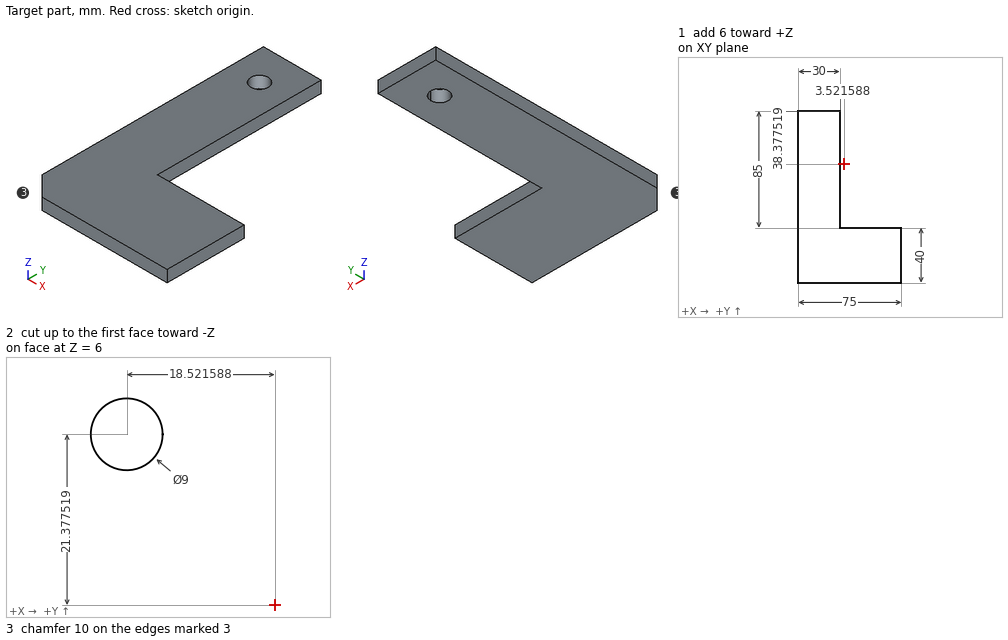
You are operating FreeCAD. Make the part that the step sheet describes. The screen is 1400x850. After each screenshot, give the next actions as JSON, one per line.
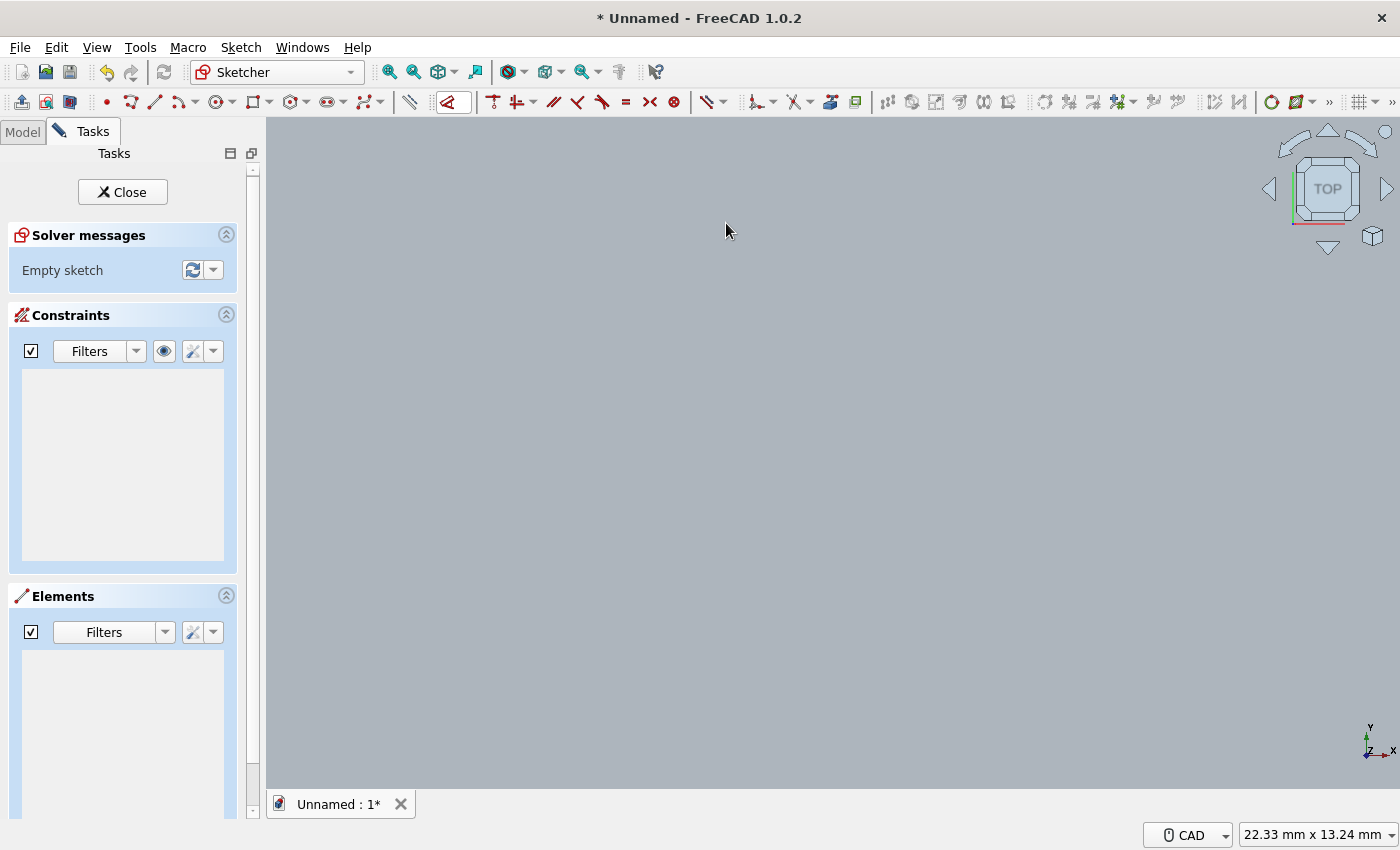
{"action": "left_click", "coordinate": [216, 102]}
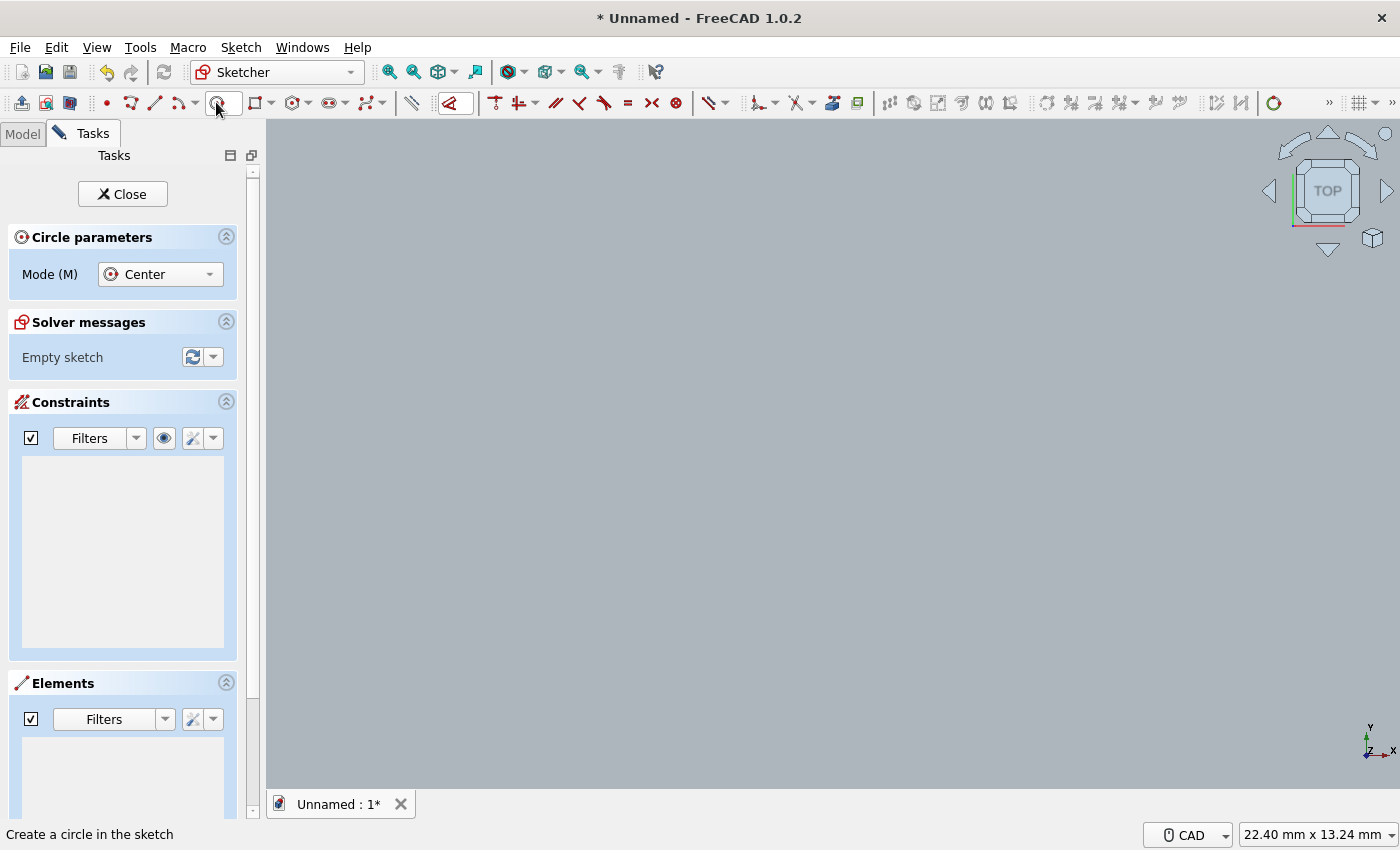
{"action": "left_click", "coordinate": [759, 448]}
{"action": "left_click", "coordinate": [920, 287]}
{"action": "key", "text": "Escape"}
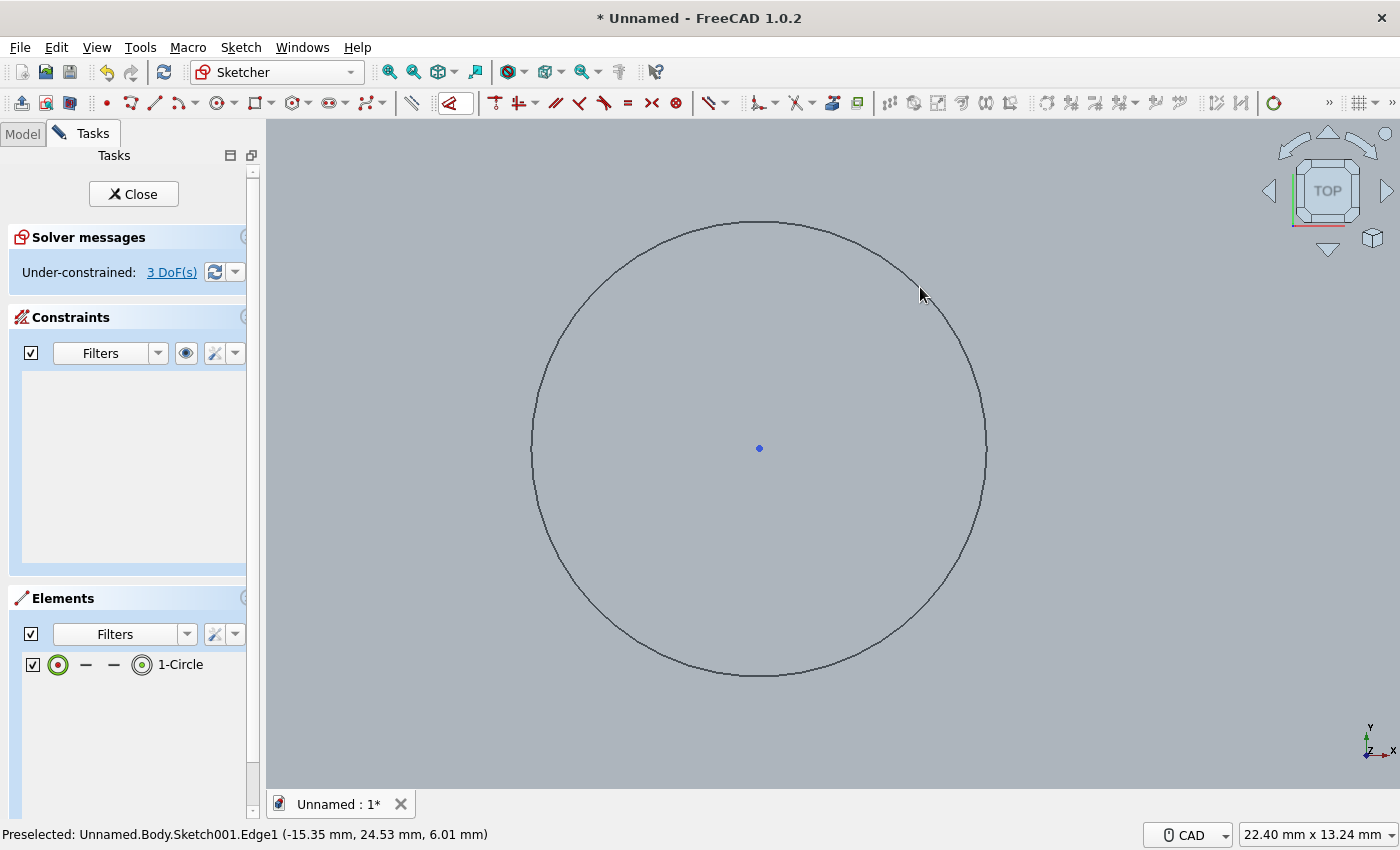
{"action": "left_click", "coordinate": [920, 288]}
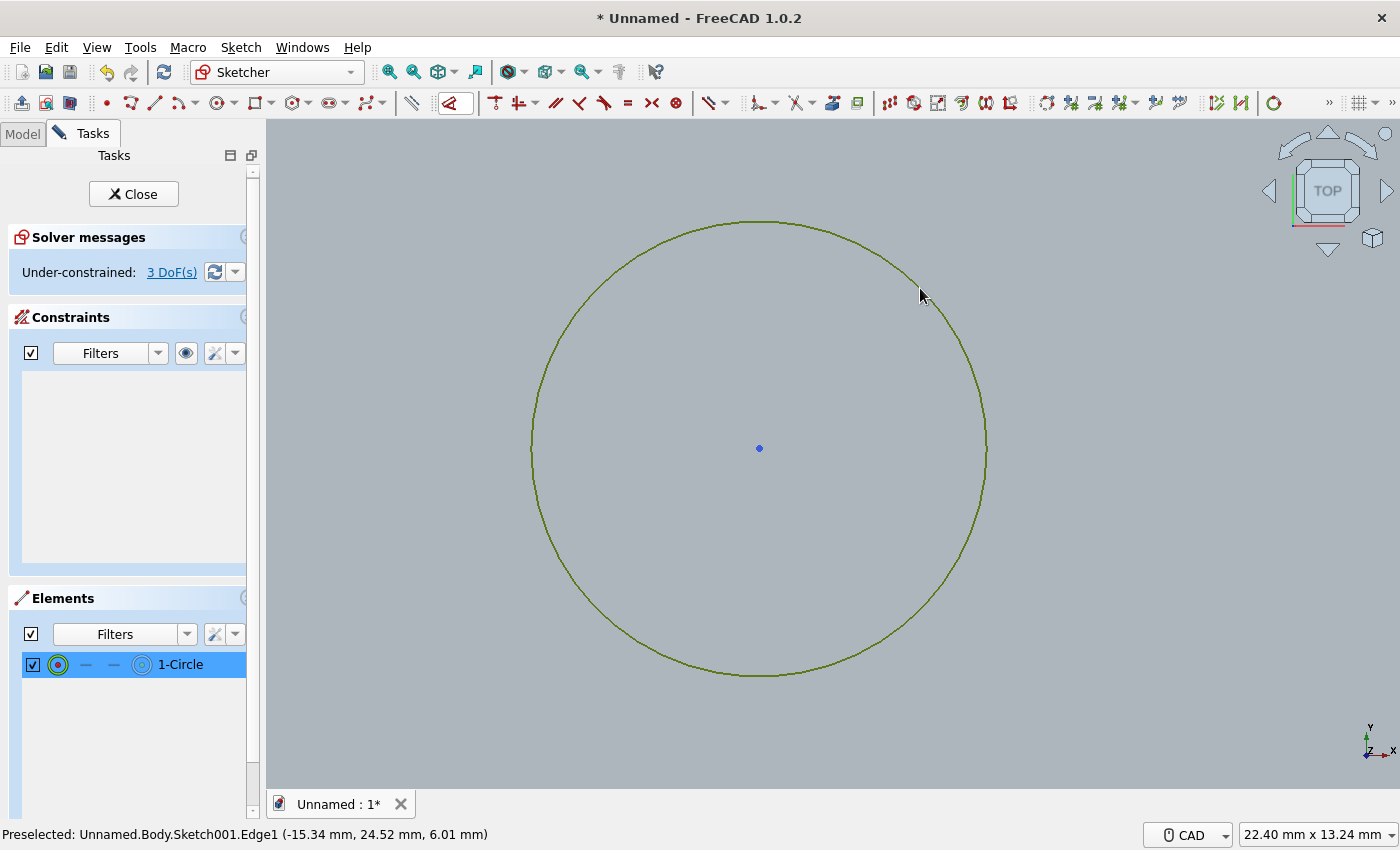
{"action": "key", "text": "k o"}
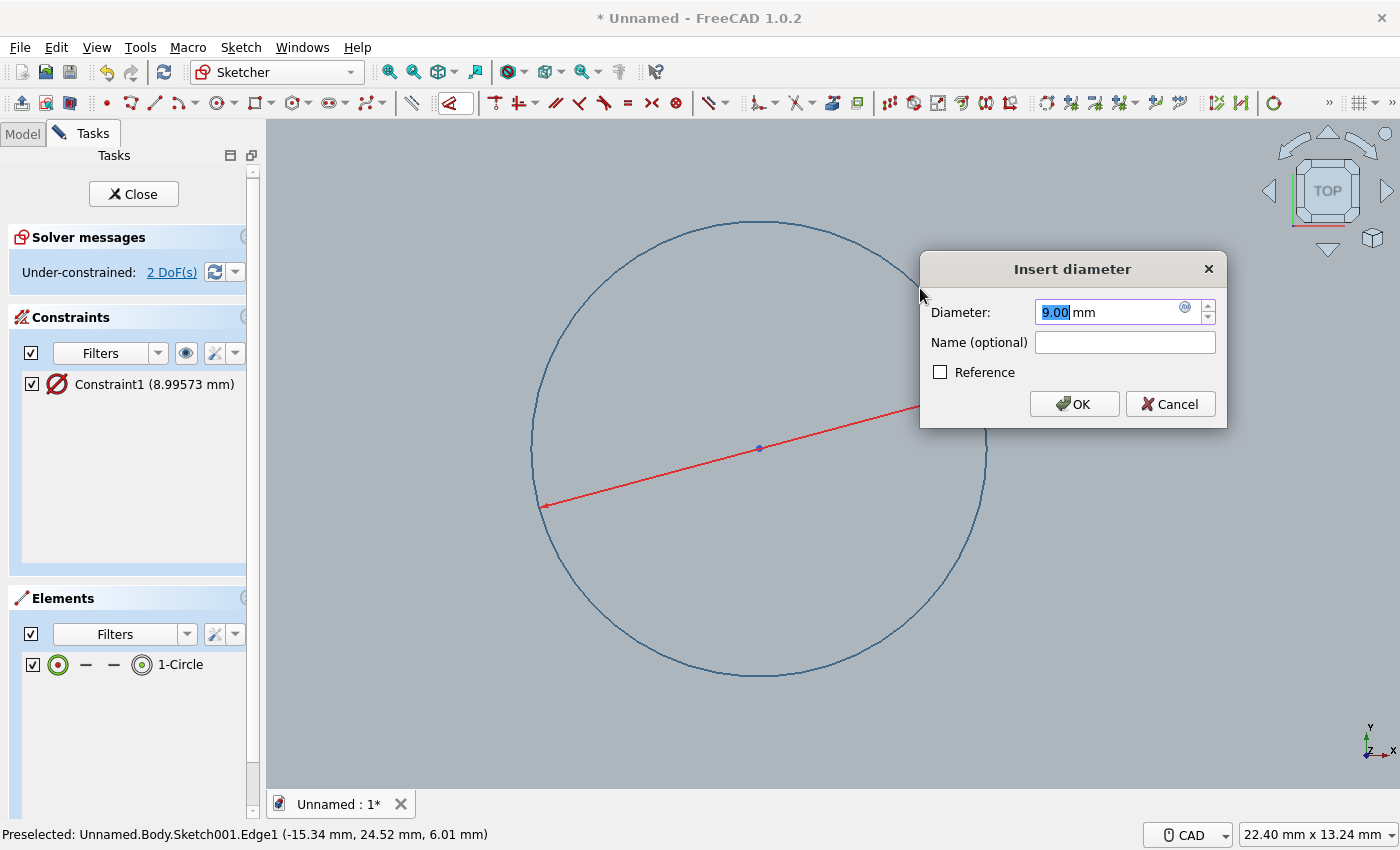
{"action": "type", "text": "9"}
{"action": "key", "text": "Return"}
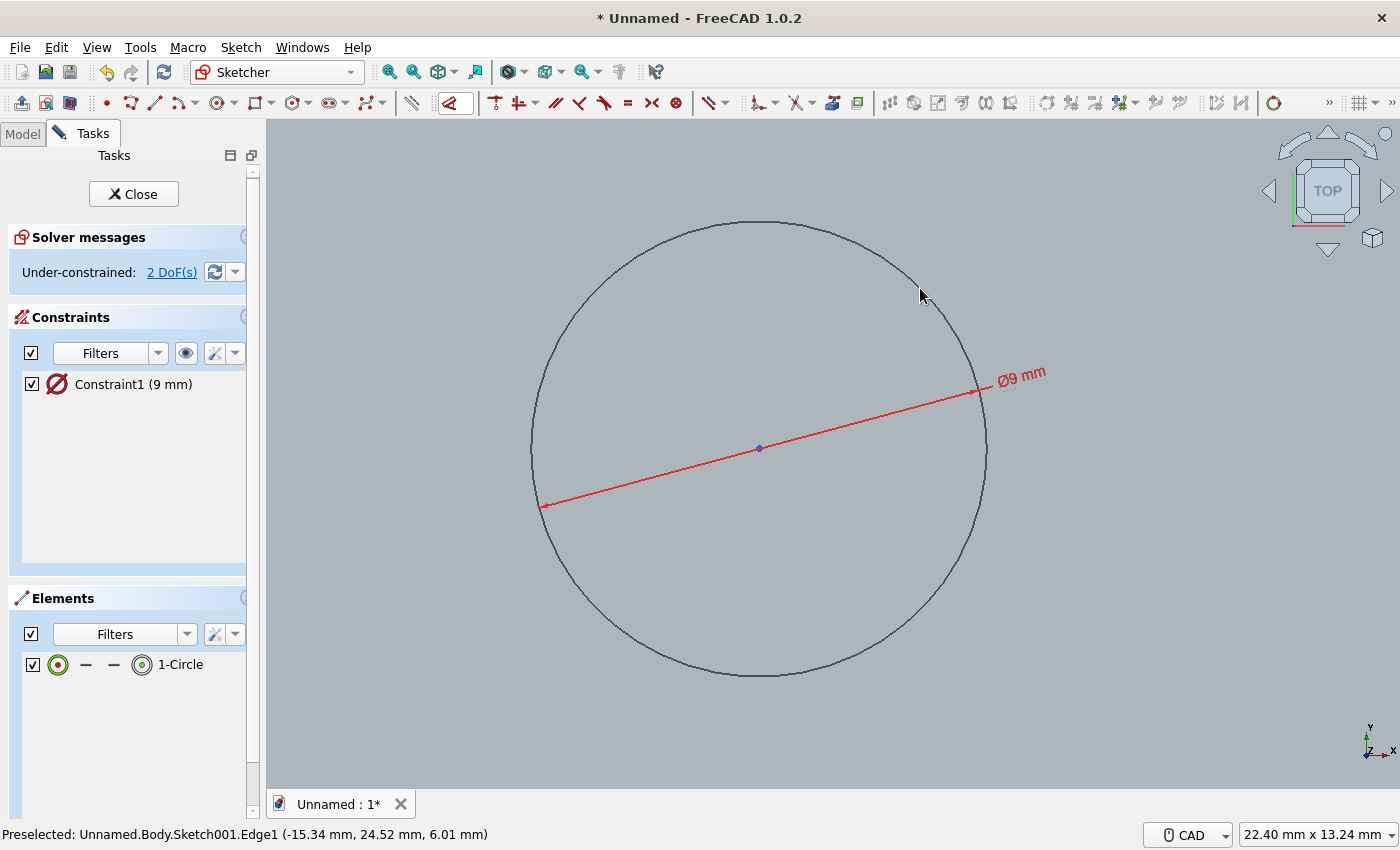
{"action": "left_click", "coordinate": [759, 449]}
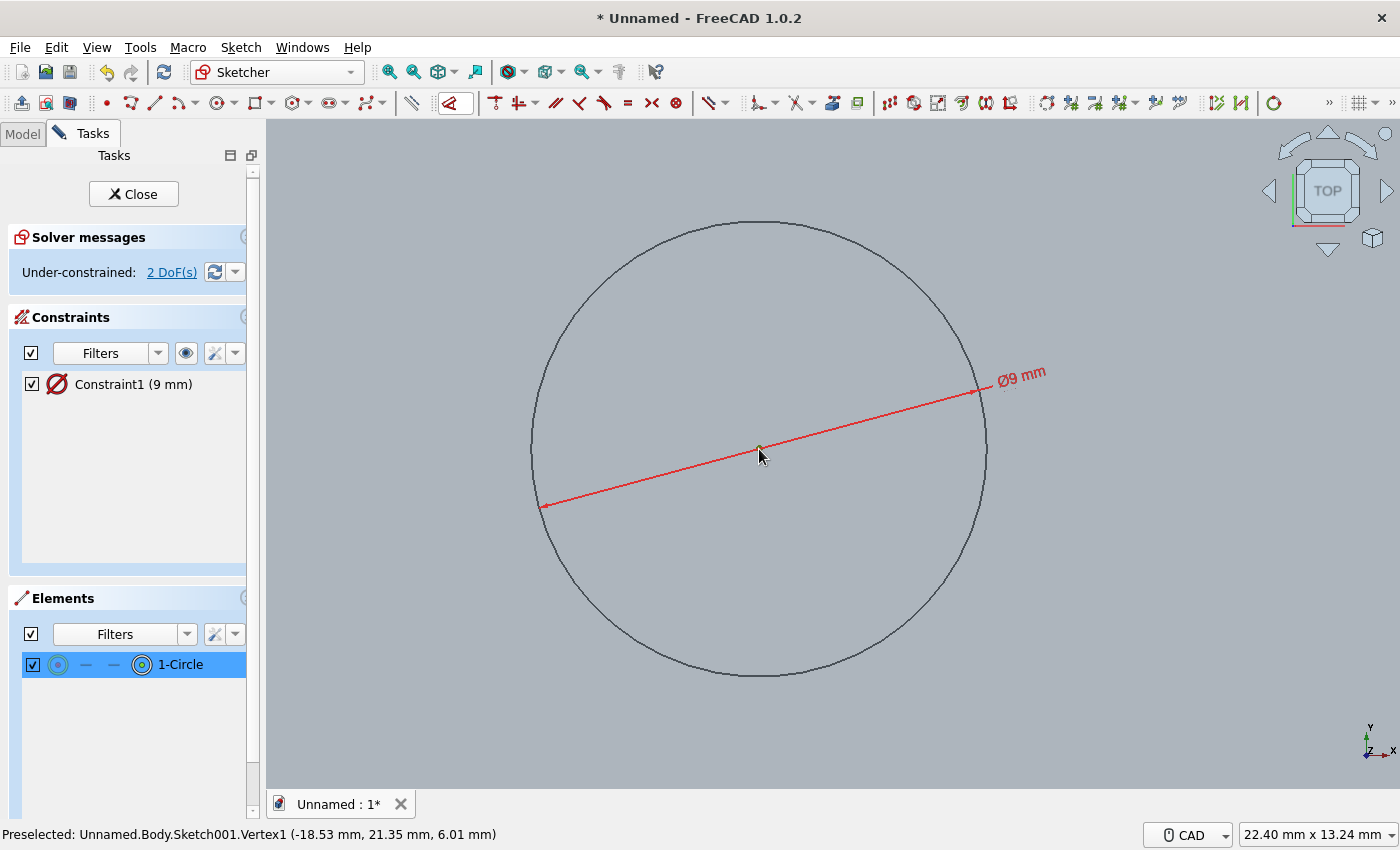
{"action": "left_click", "coordinate": [468, 104]}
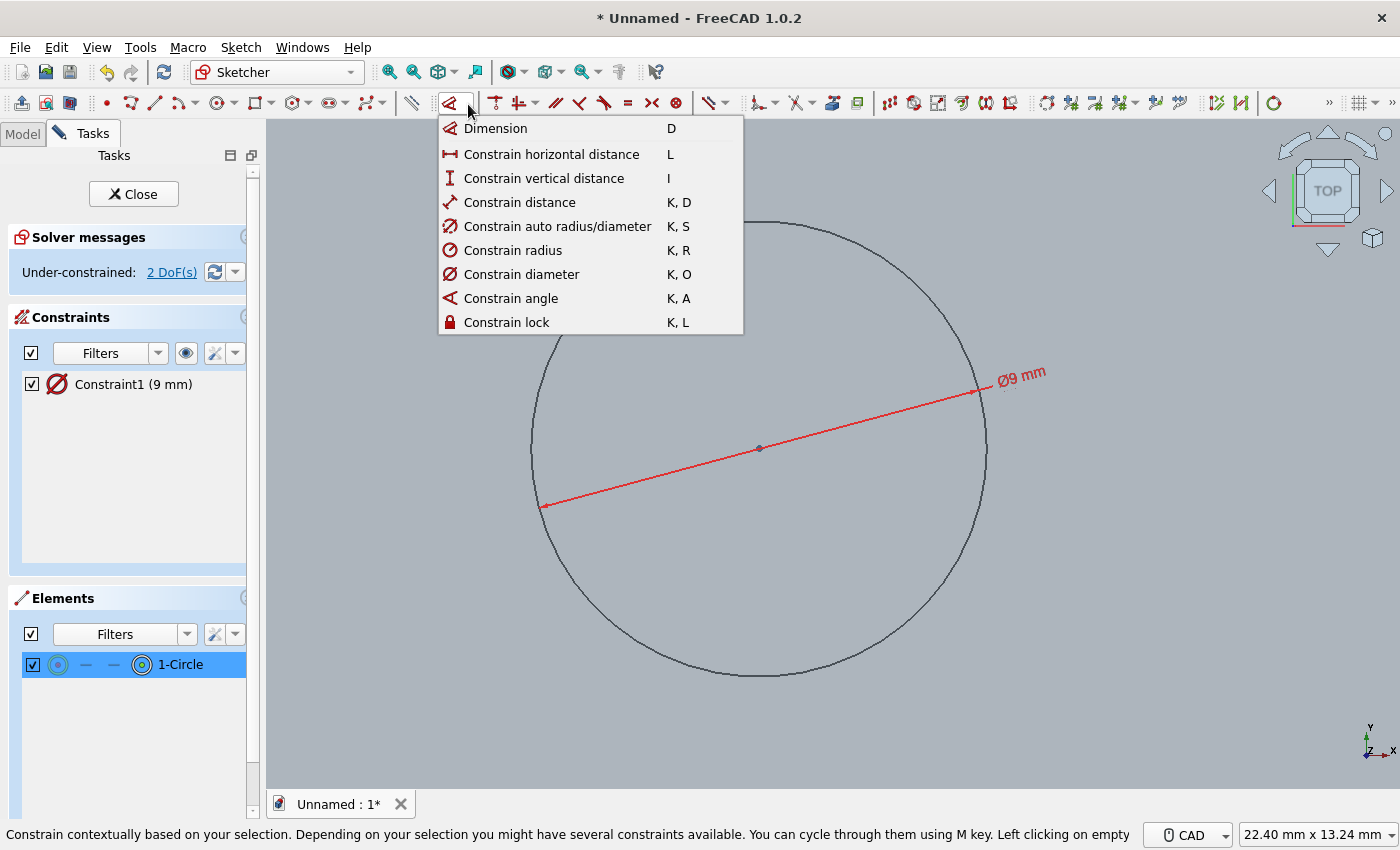
{"action": "left_click", "coordinate": [591, 154]}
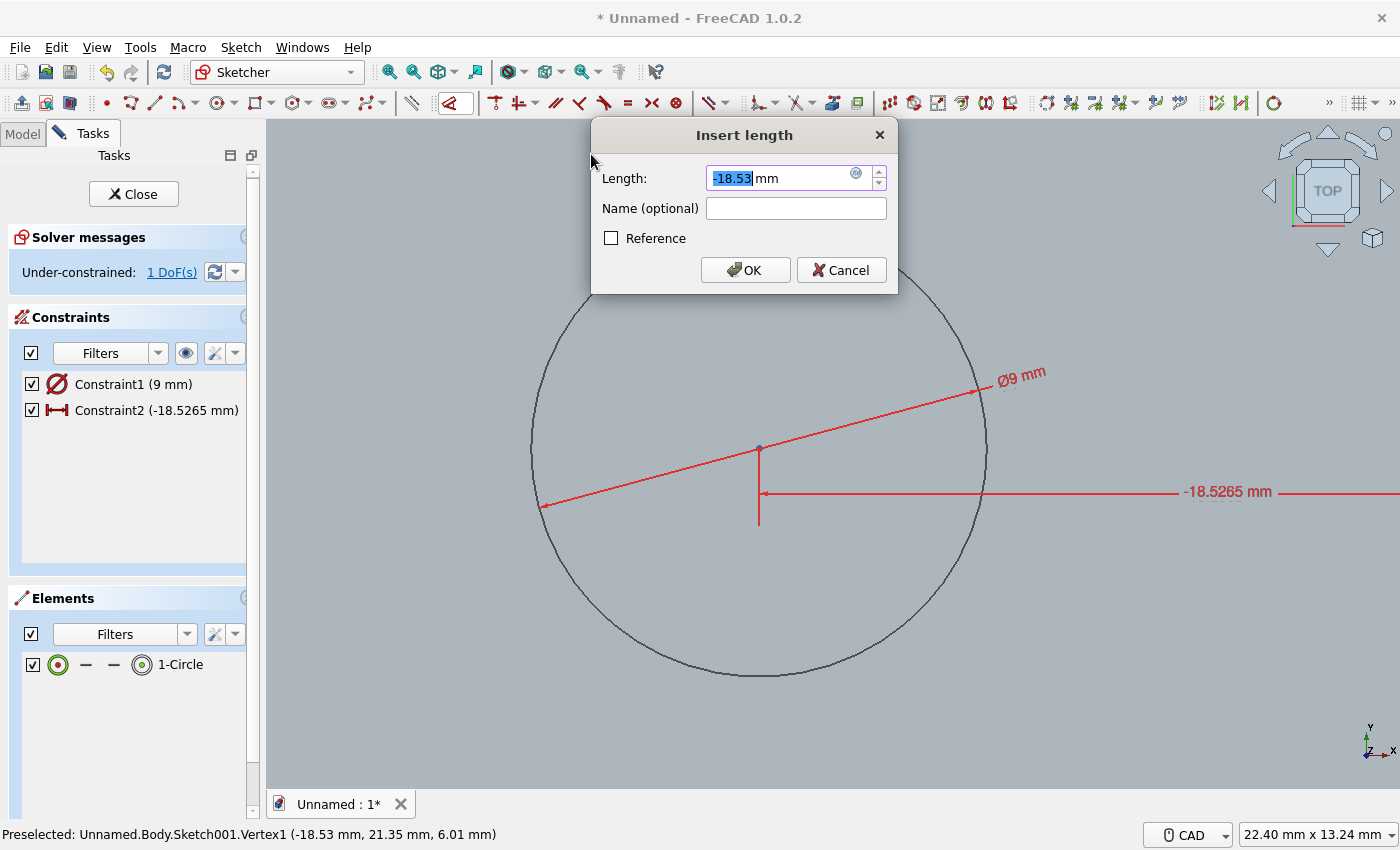
{"action": "type", "text": "-18.521588"}
{"action": "key", "text": "Return"}